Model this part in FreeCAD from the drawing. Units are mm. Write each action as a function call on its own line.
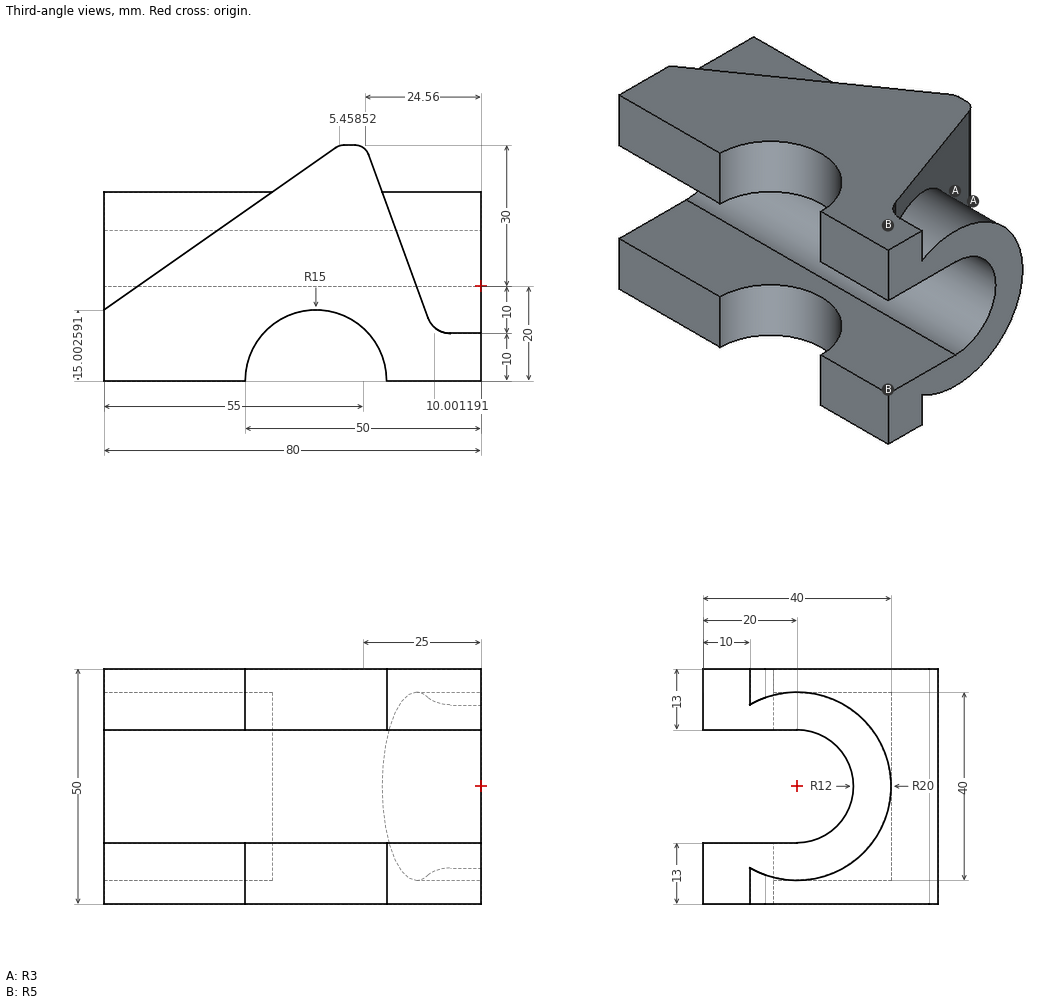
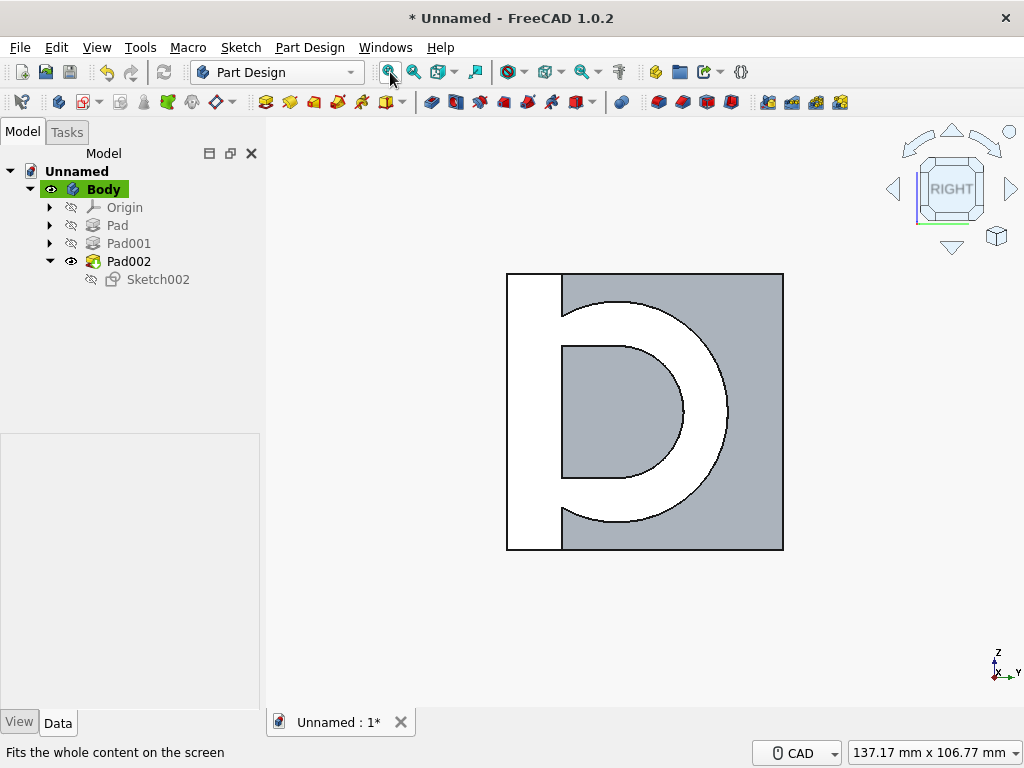
key(5)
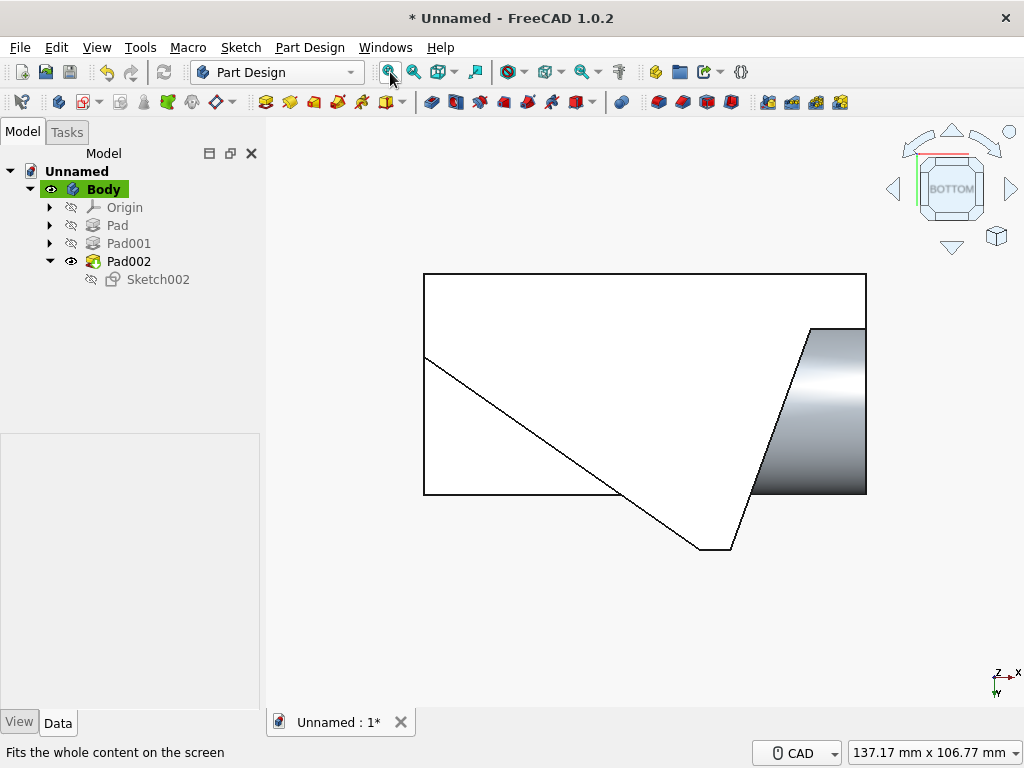
key(4)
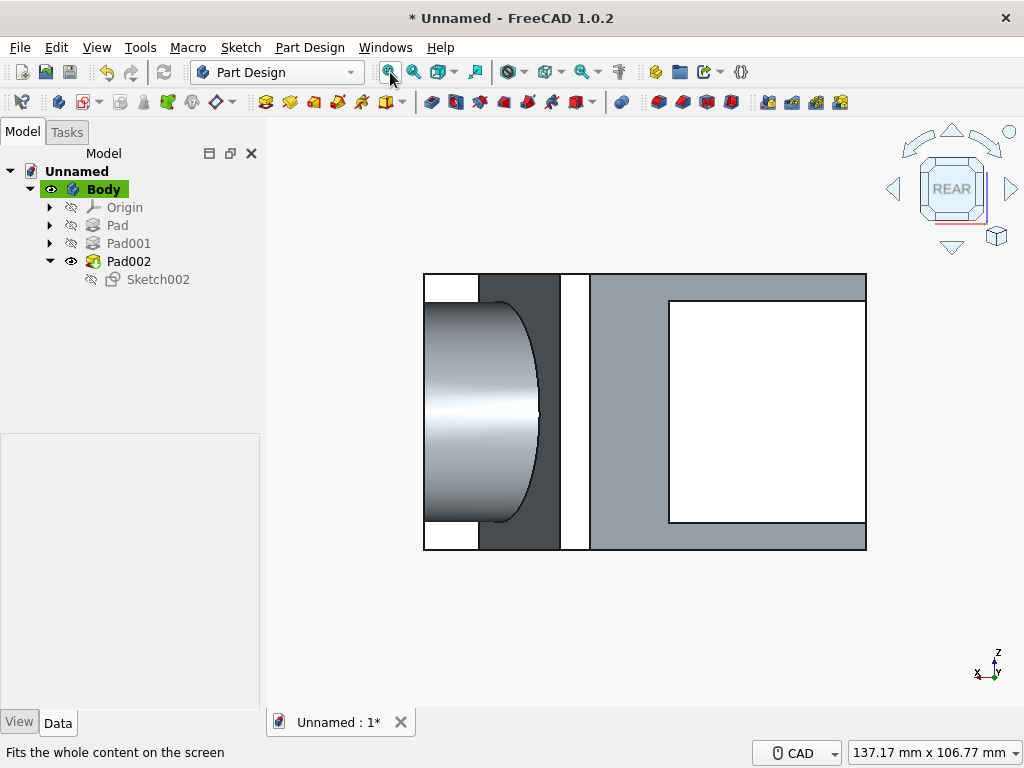
click(590, 411)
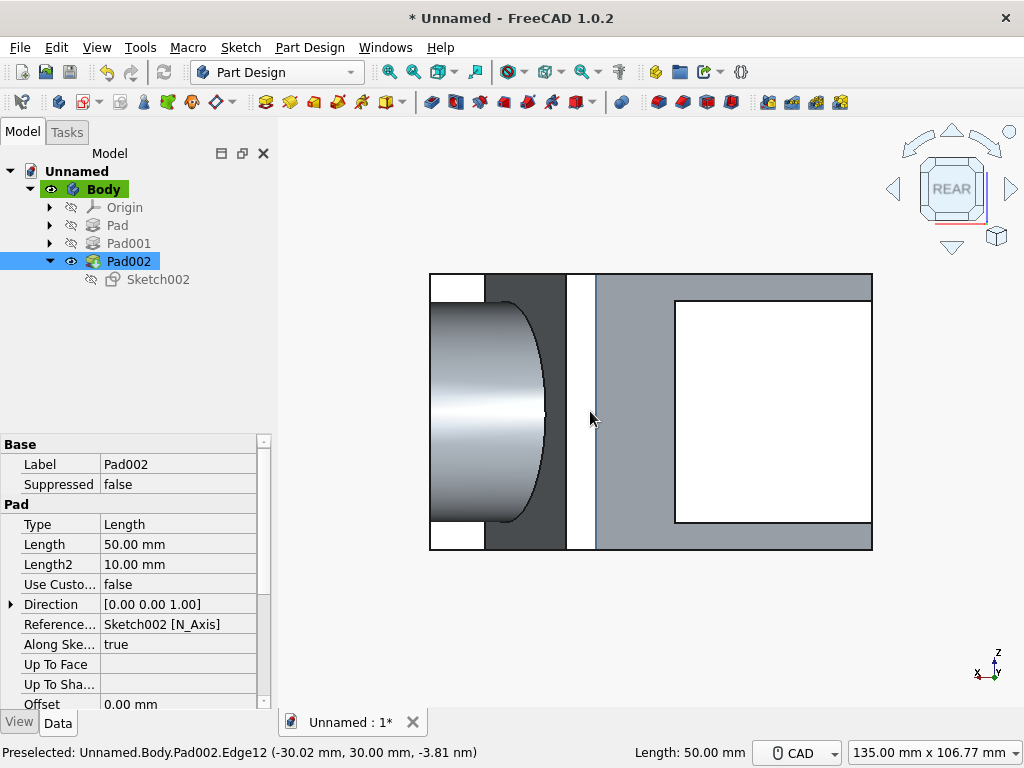
click(566, 411, ctrl)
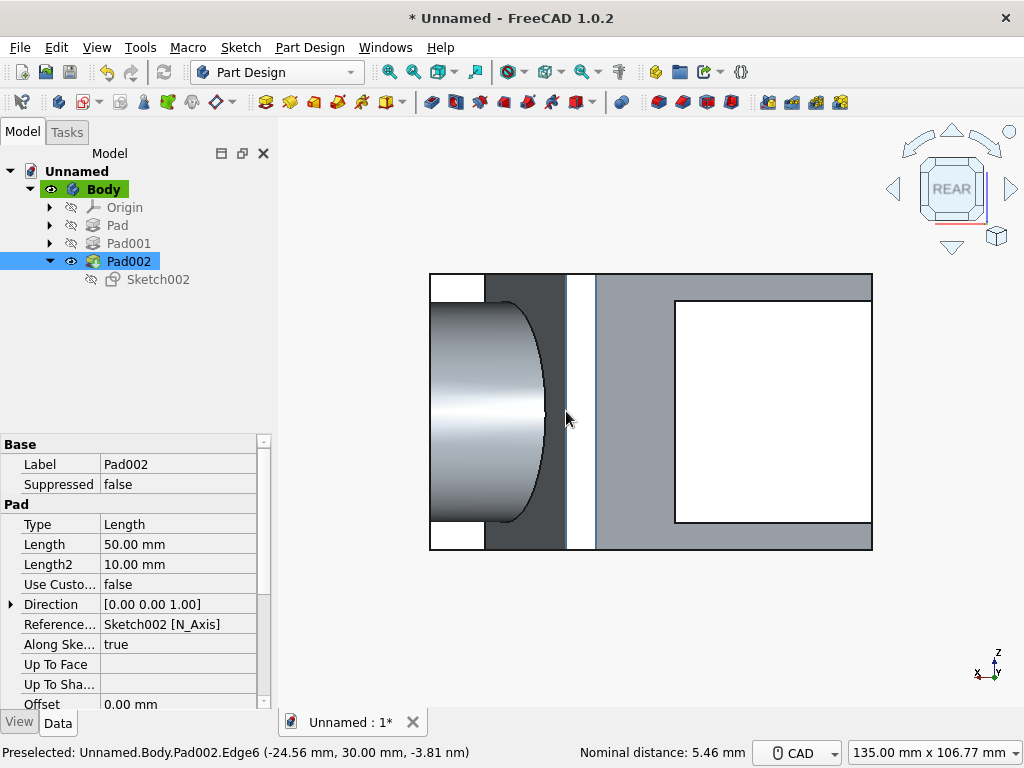
click(660, 102)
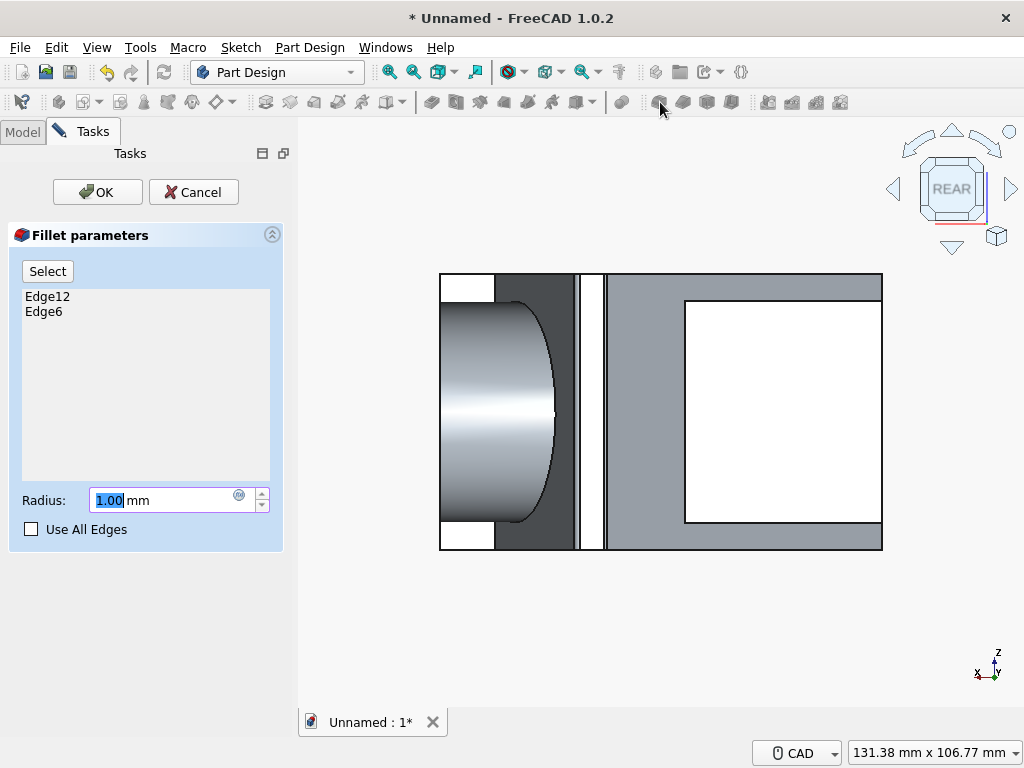
text(3)
key(Tab)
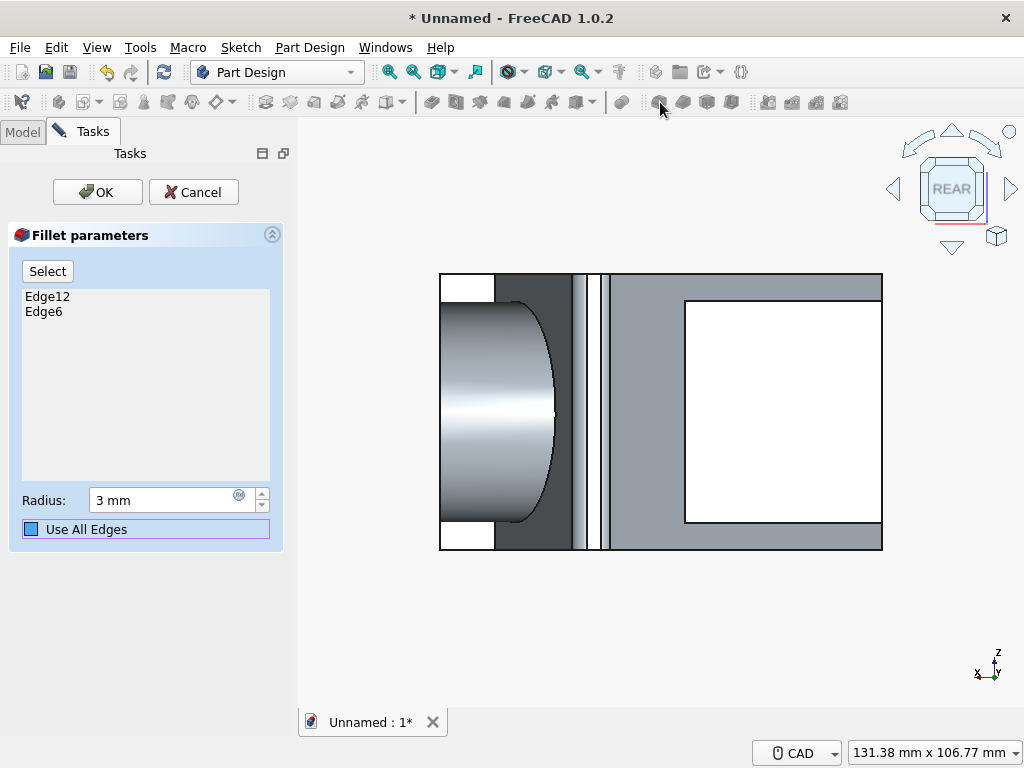
click(98, 192)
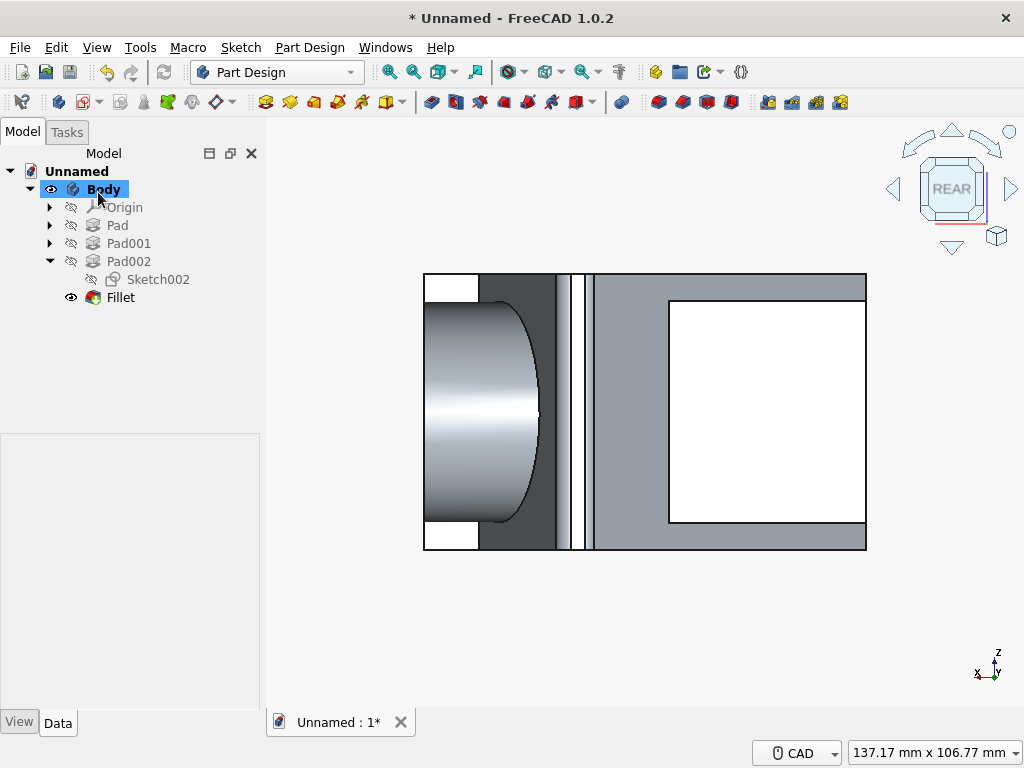
click(84, 102)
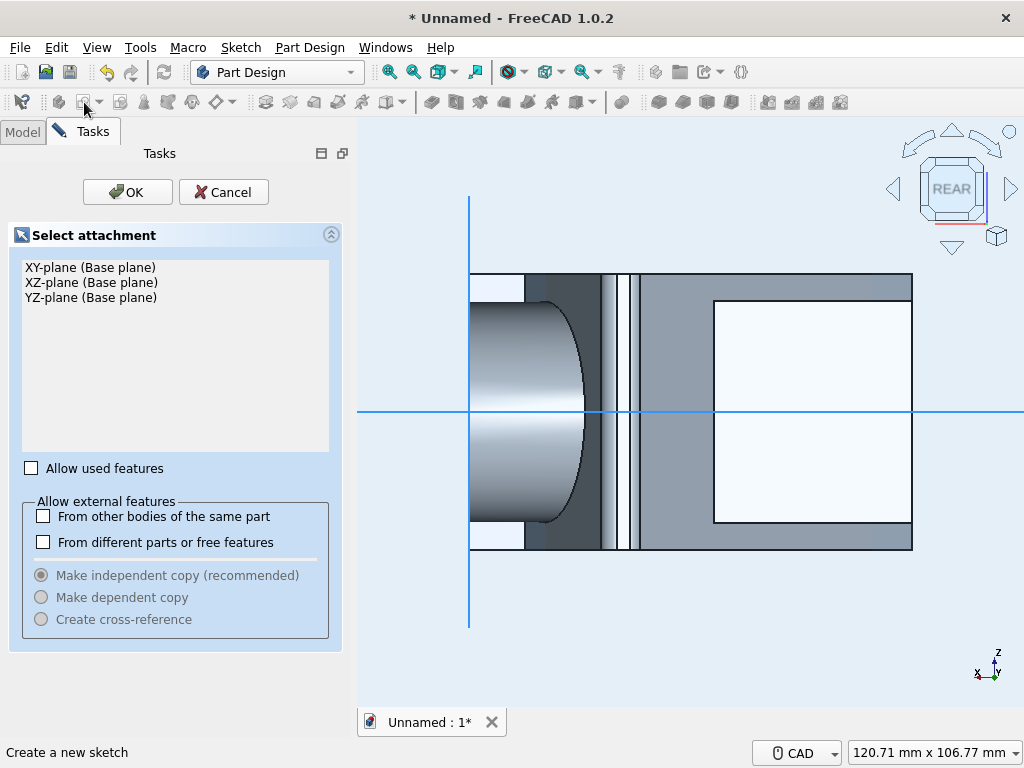
click(82, 298)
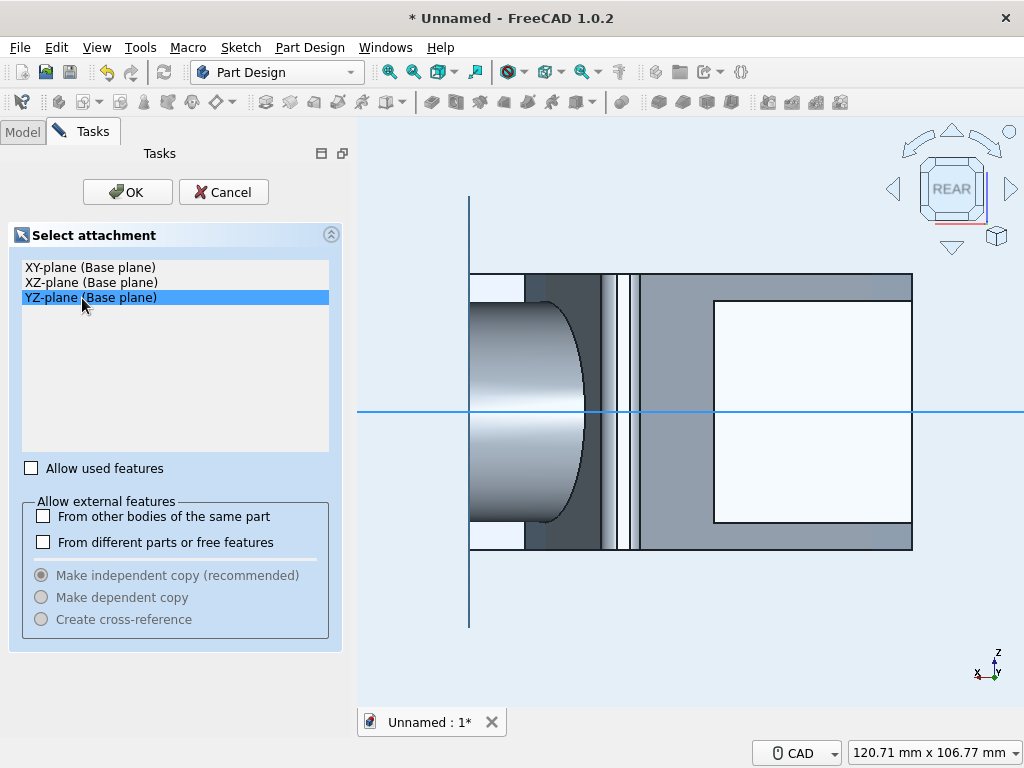
click(128, 192)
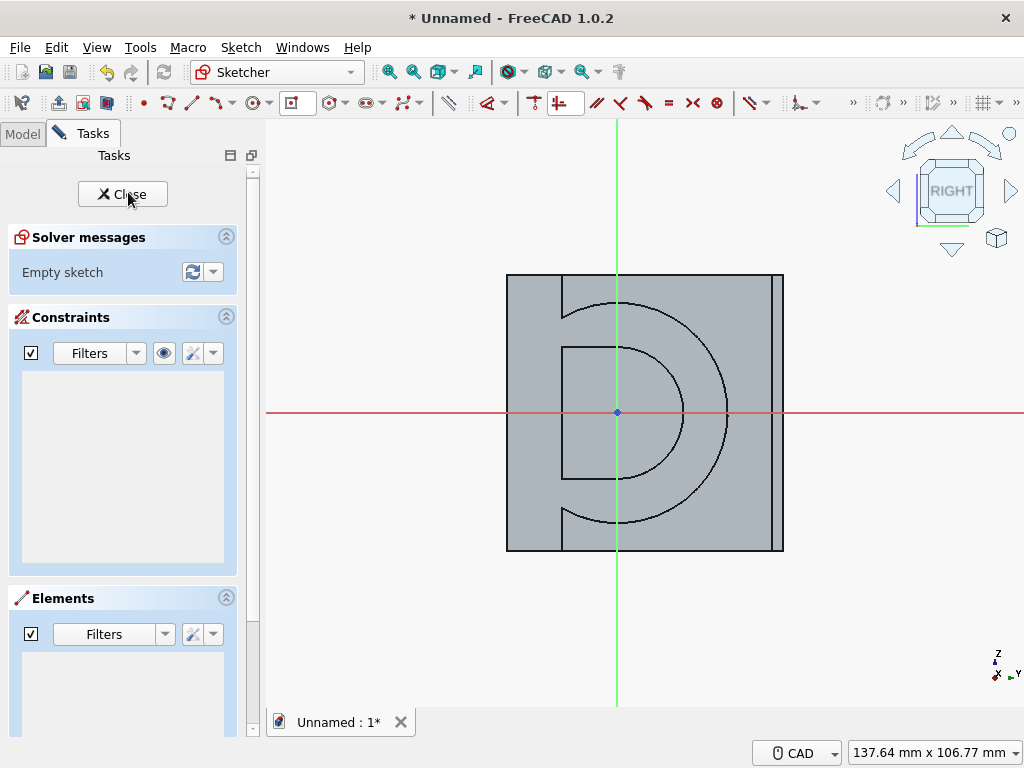
scroll(611, 413, up, 4)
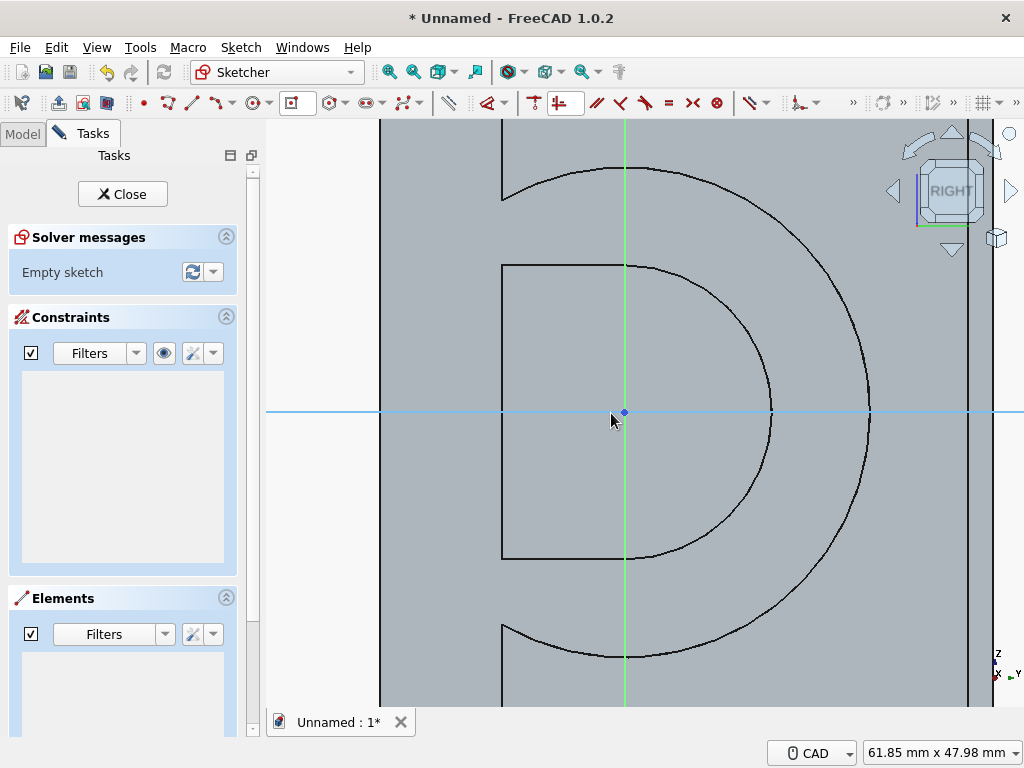
click(168, 104)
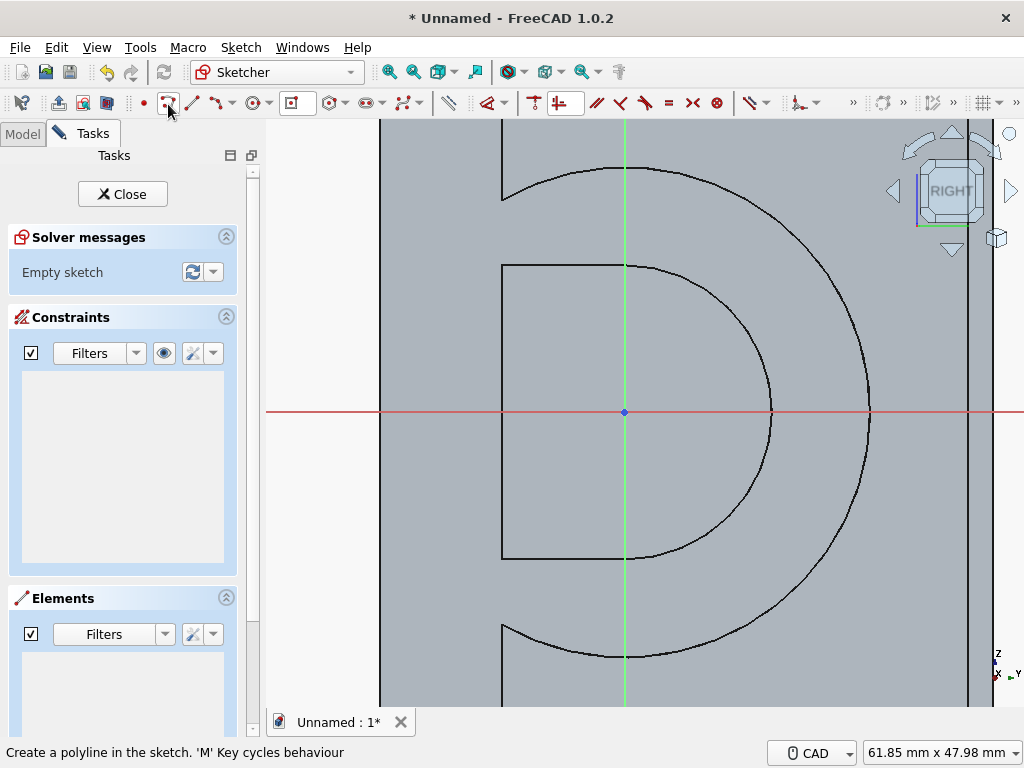
click(625, 265)
click(380, 265)
click(380, 559)
click(625, 559)
right_click(625, 559)